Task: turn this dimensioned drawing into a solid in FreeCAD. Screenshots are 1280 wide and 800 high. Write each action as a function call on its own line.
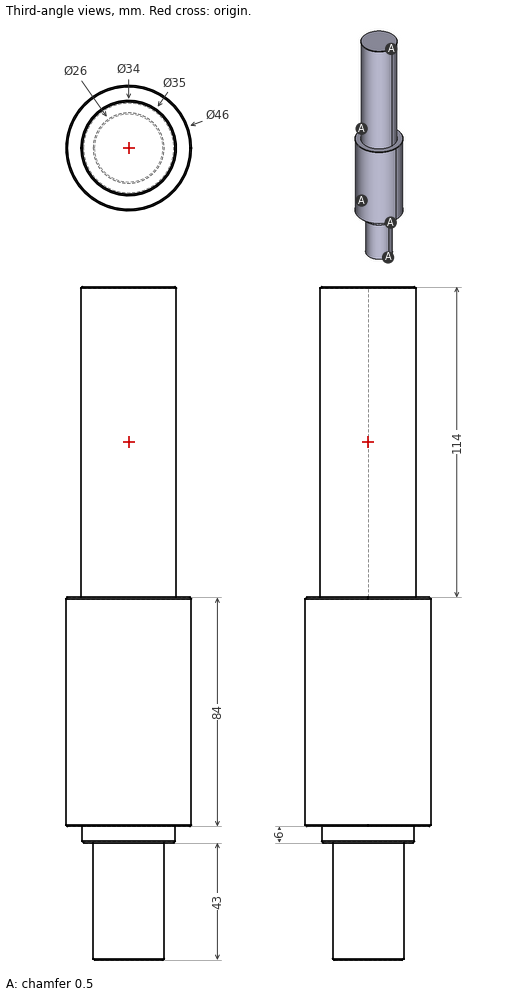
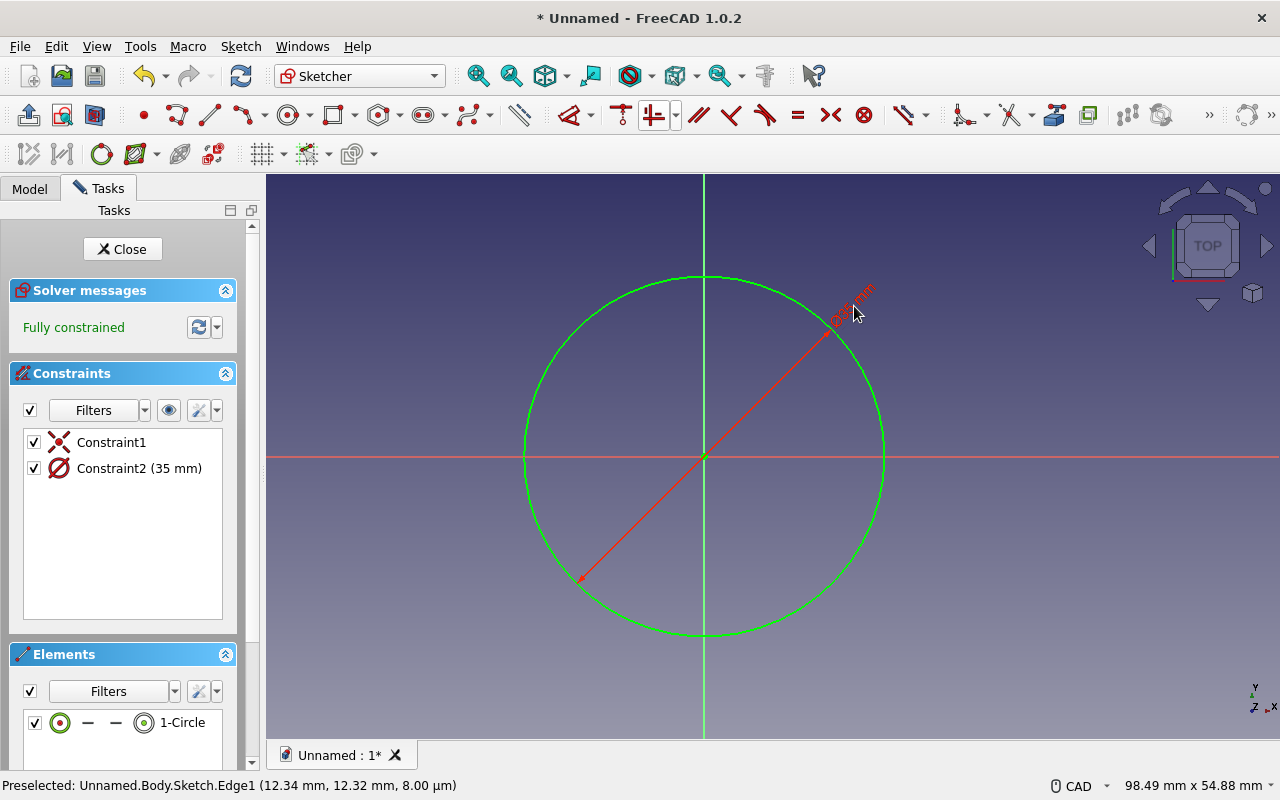
click(123, 249)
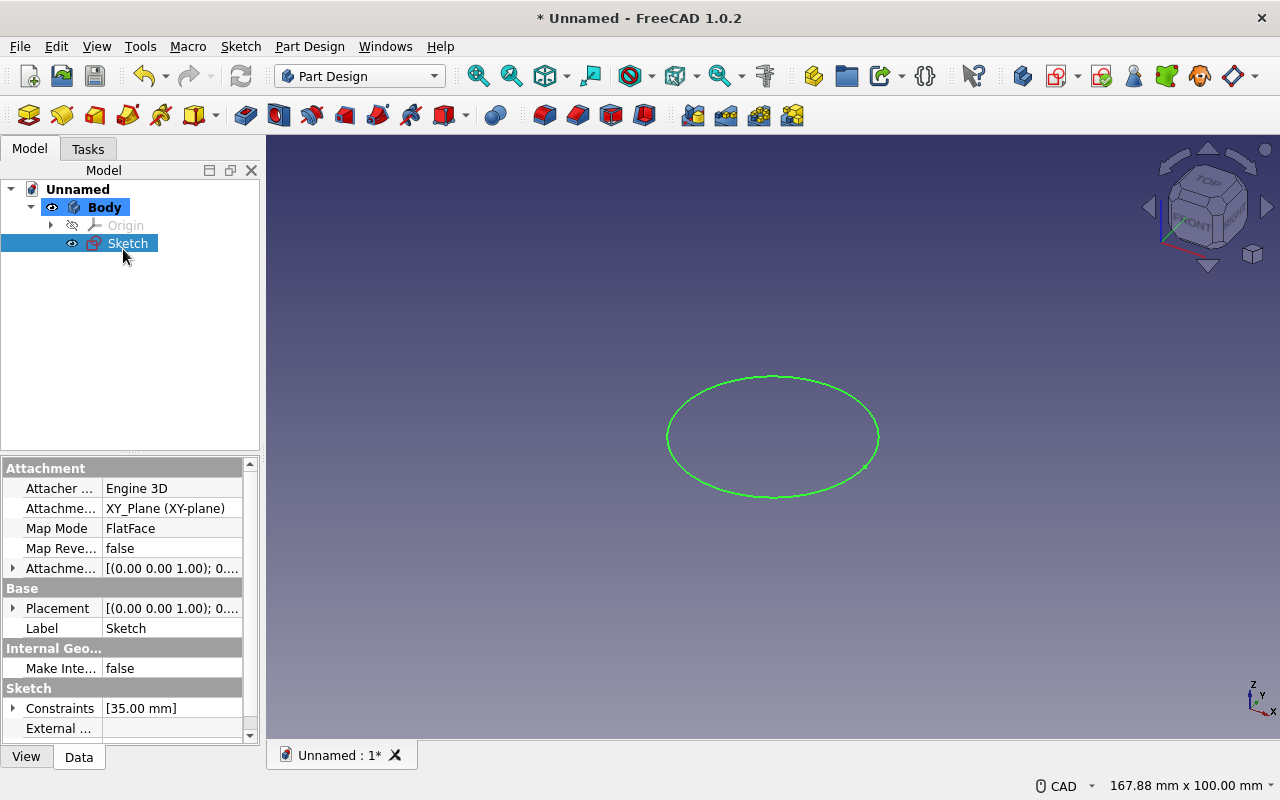
click(29, 116)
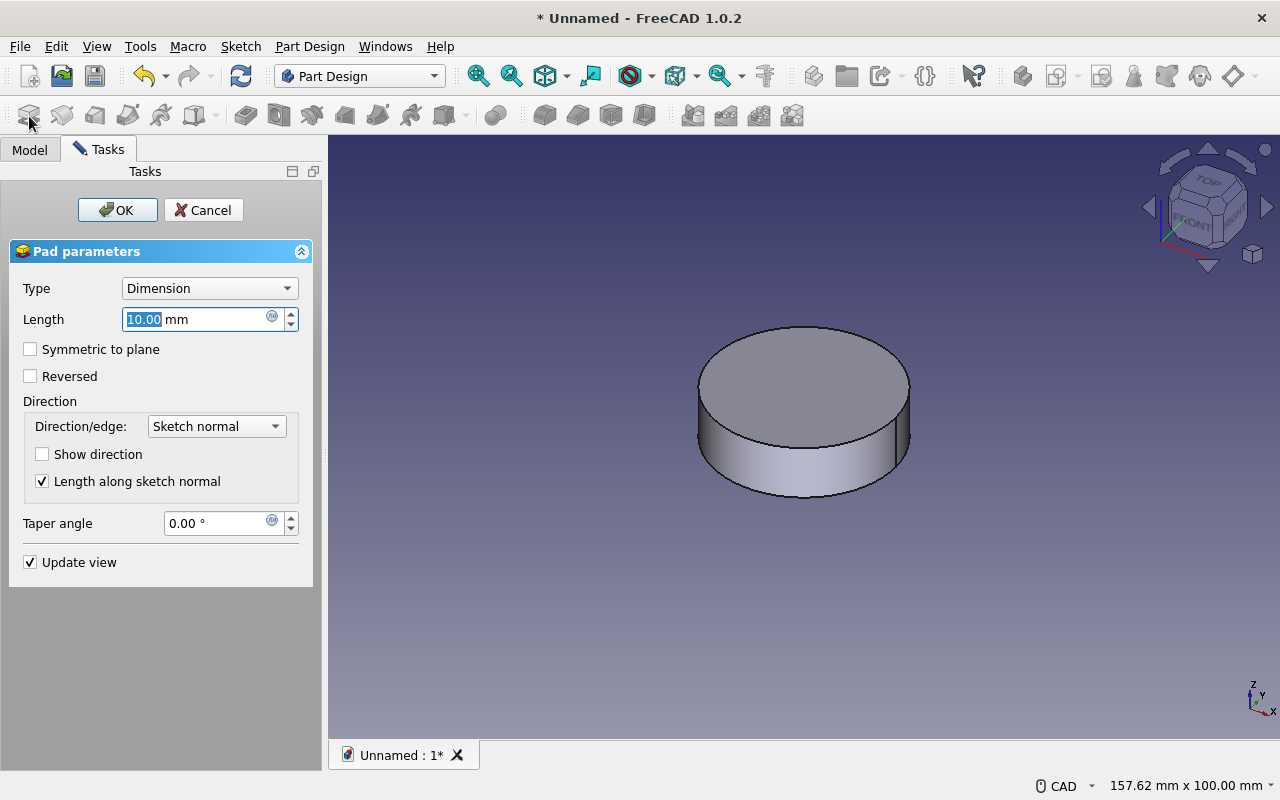
text(114)
key(Tab)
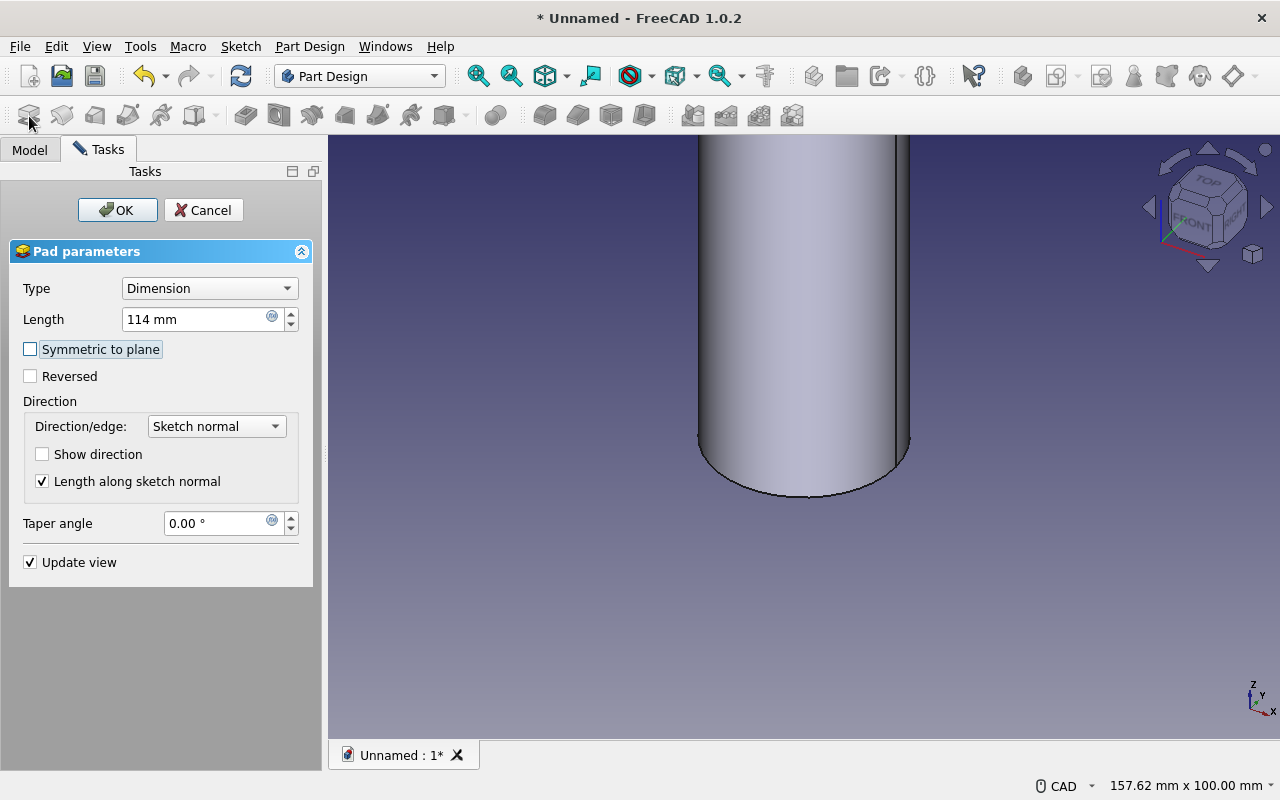
click(31, 349)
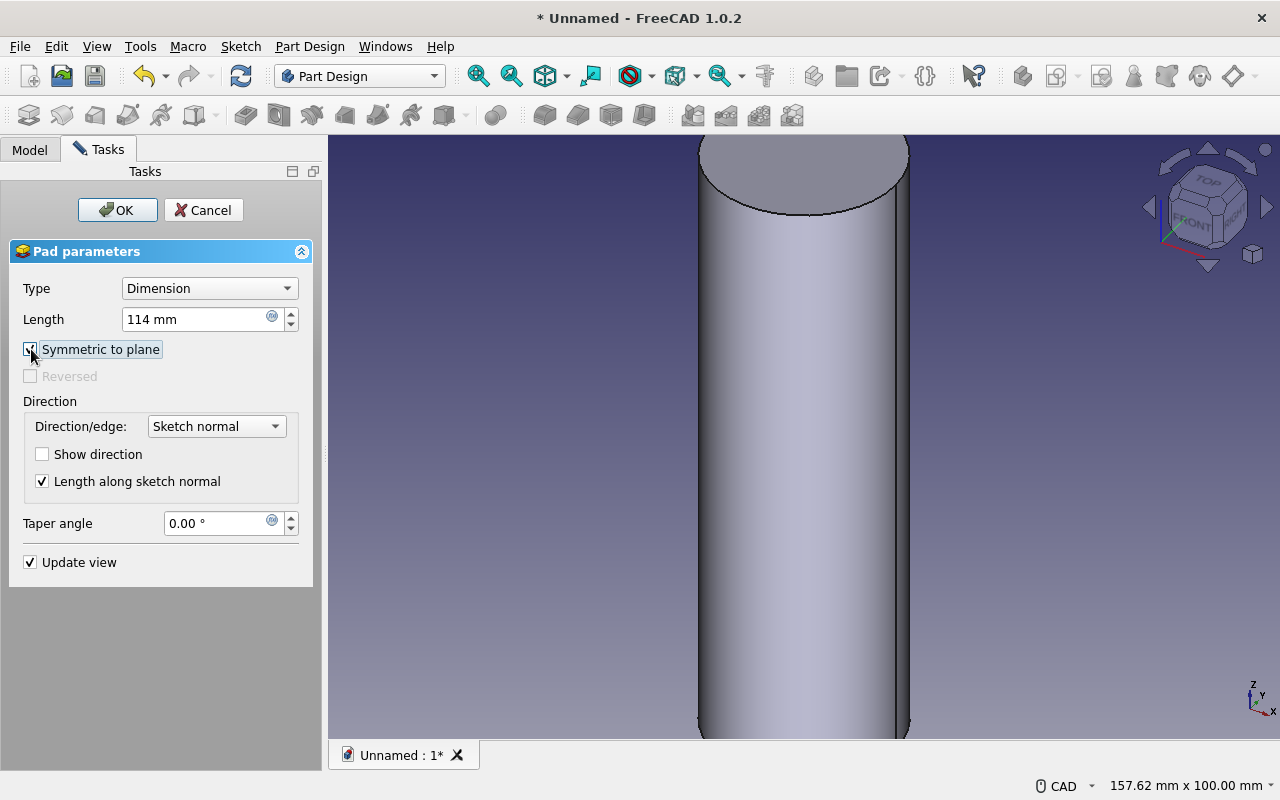
click(118, 210)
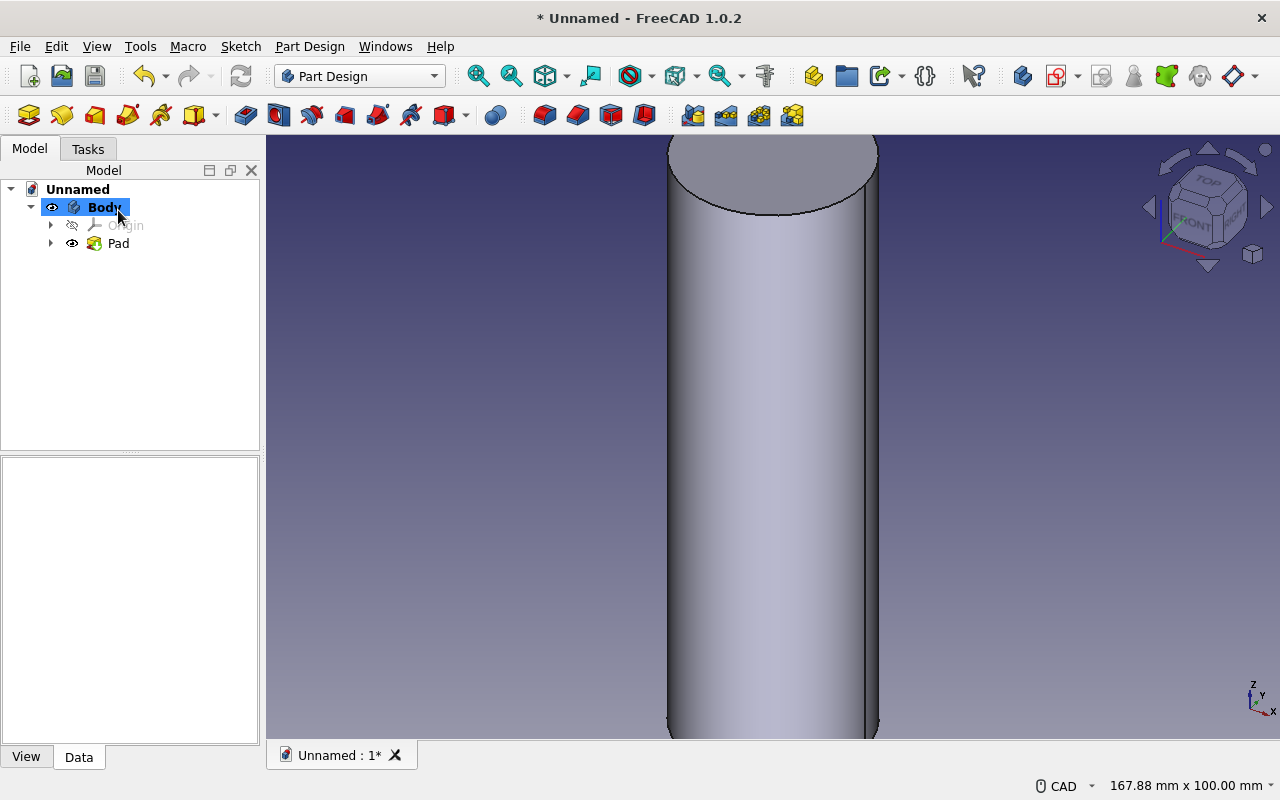
key(v)
key(f)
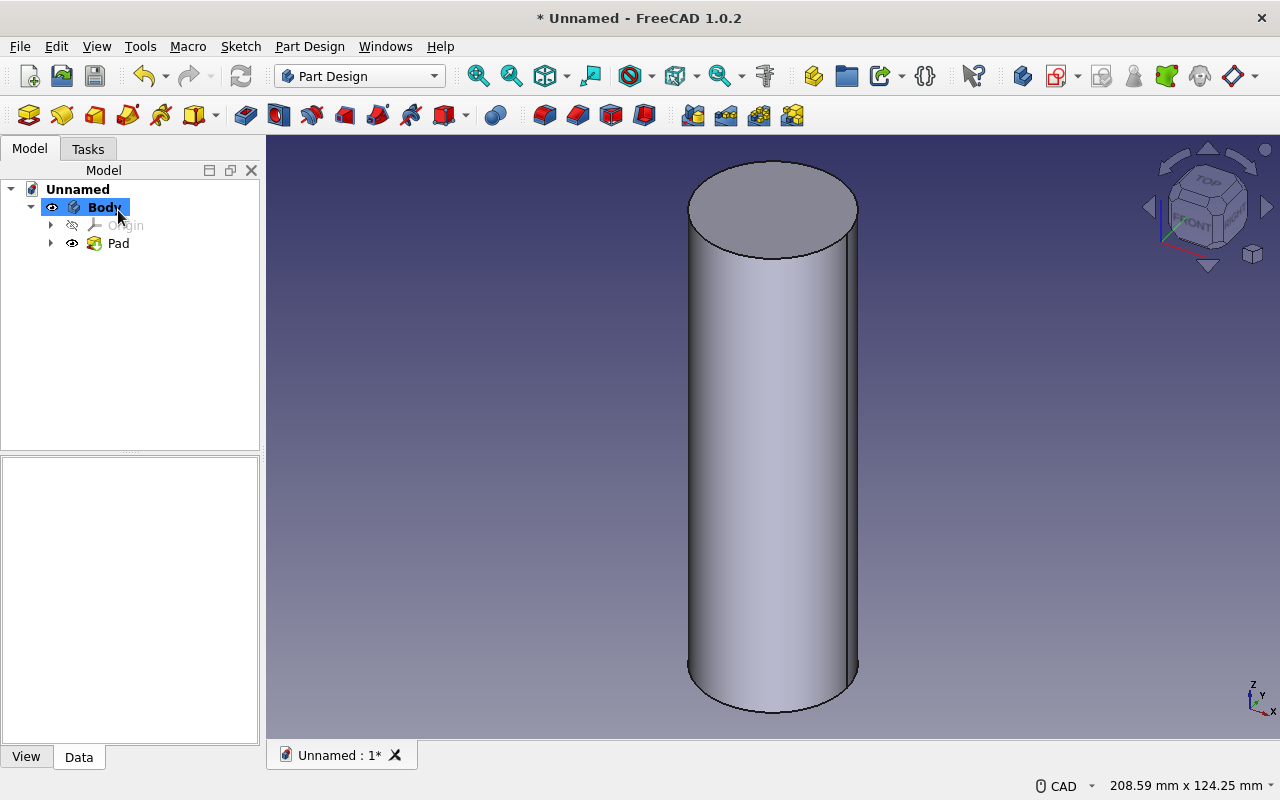
key(5)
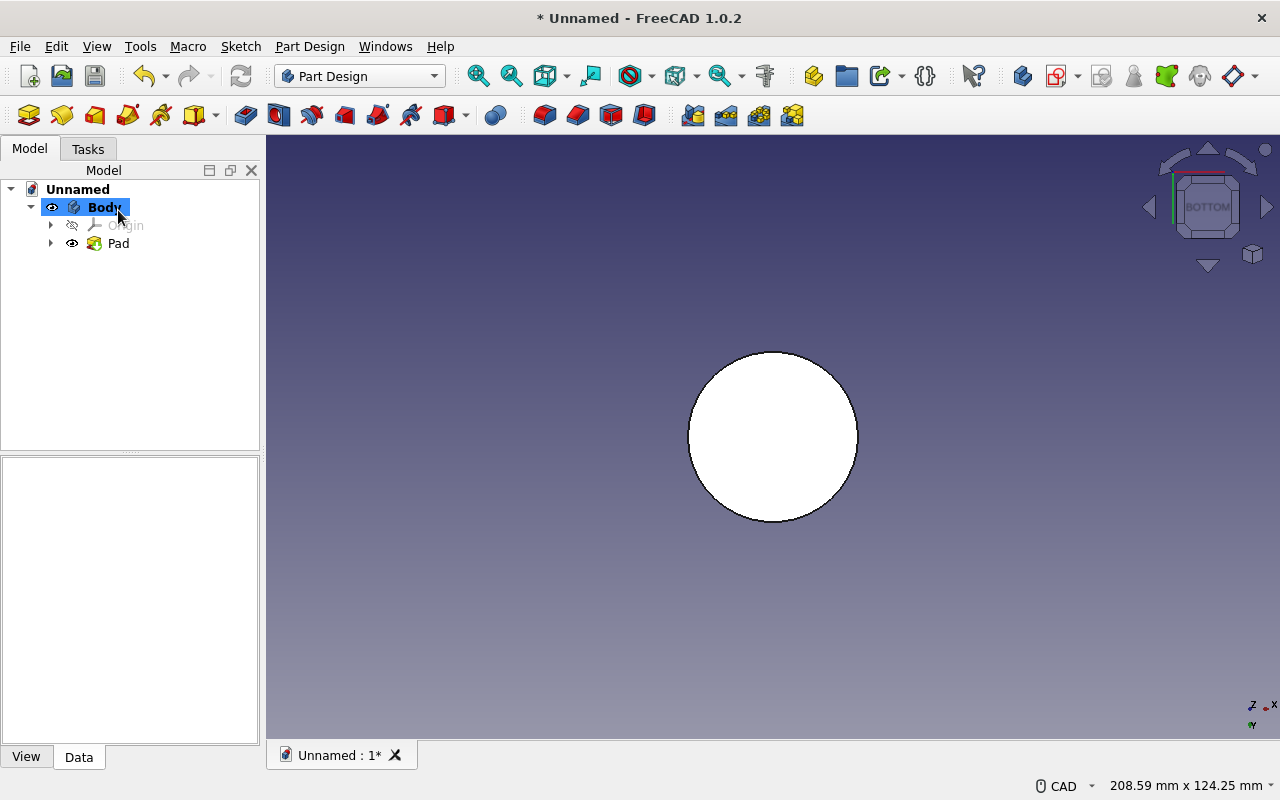
key(v)
key(f)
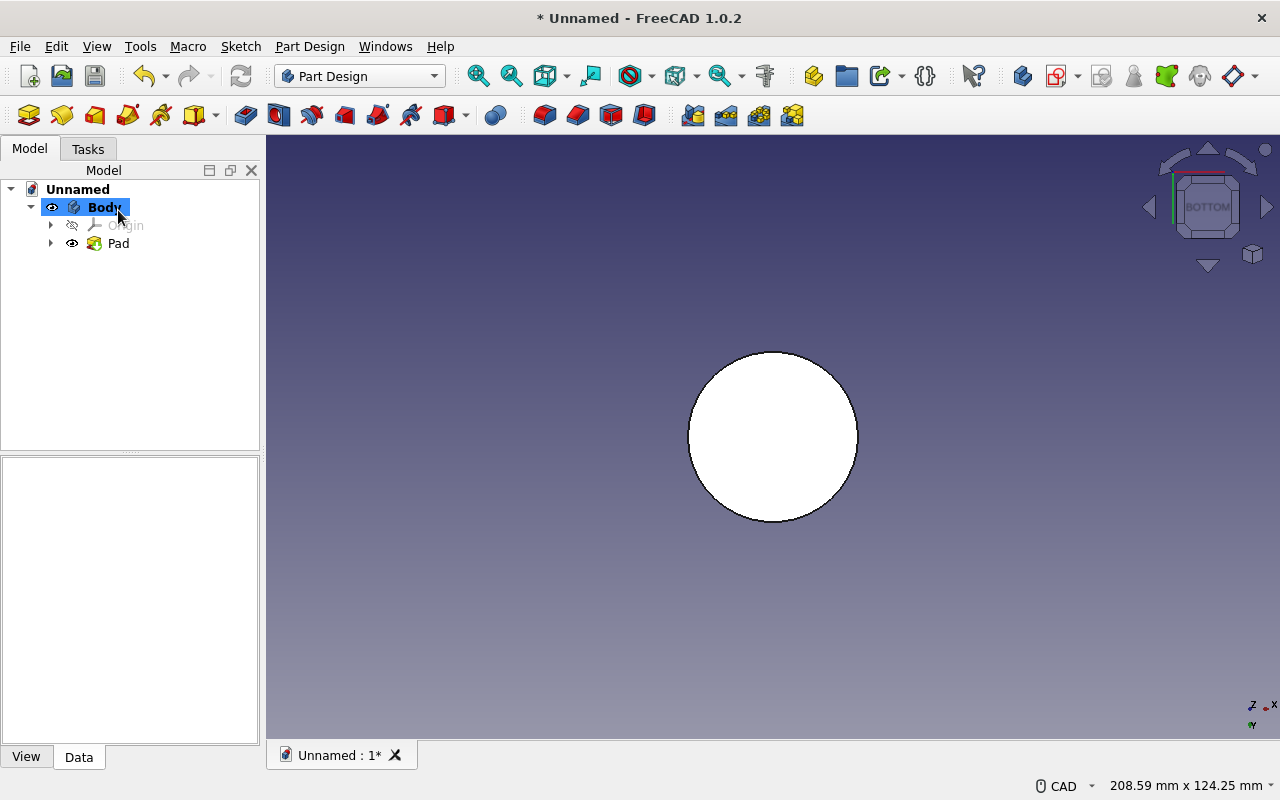
click(773, 436)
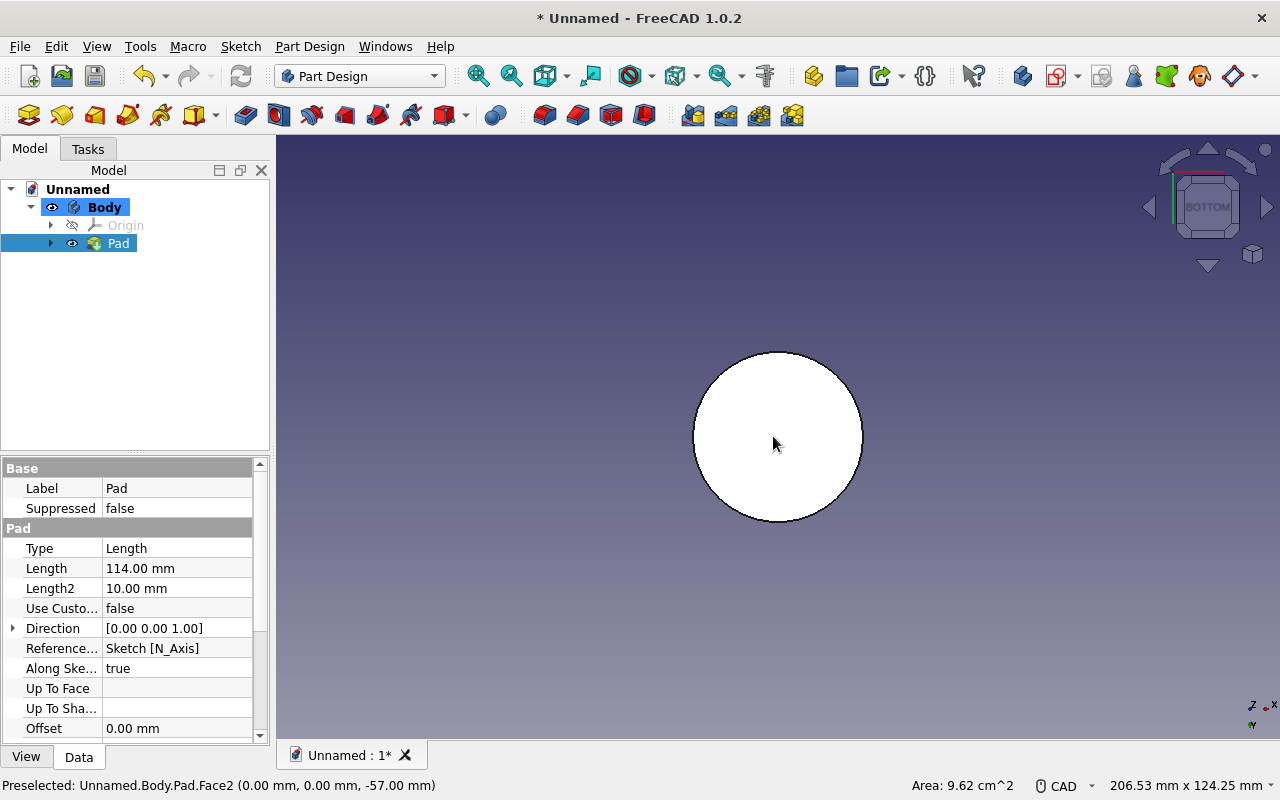
click(1056, 76)